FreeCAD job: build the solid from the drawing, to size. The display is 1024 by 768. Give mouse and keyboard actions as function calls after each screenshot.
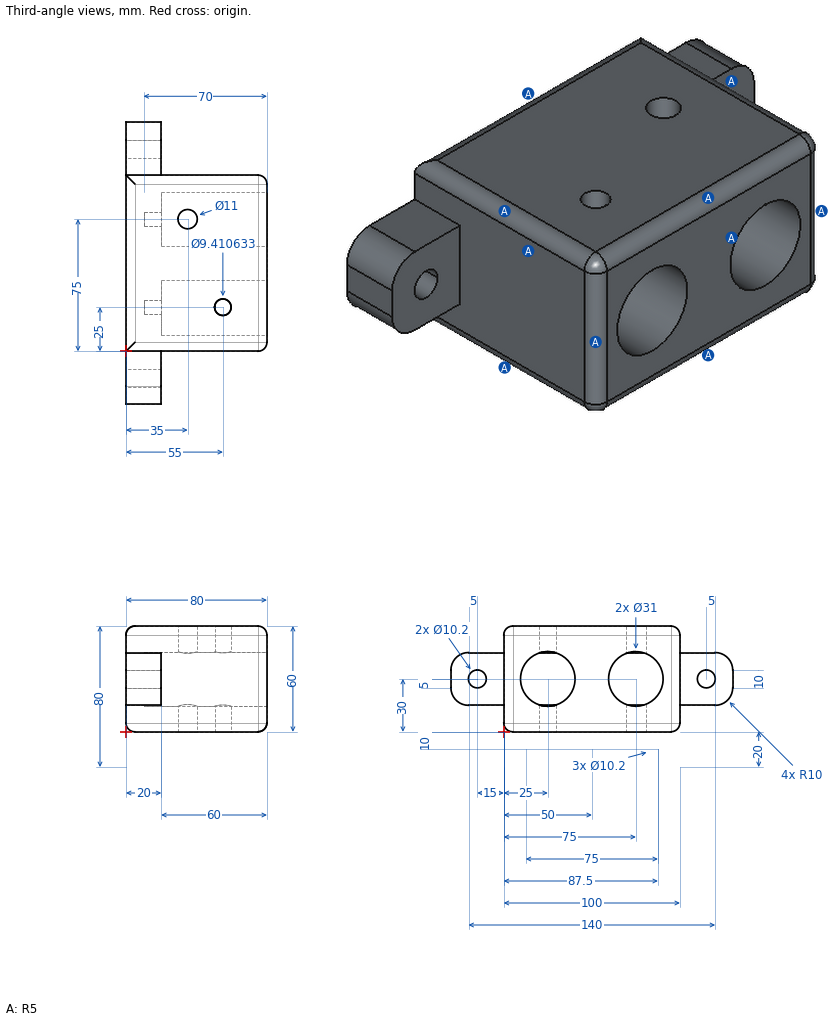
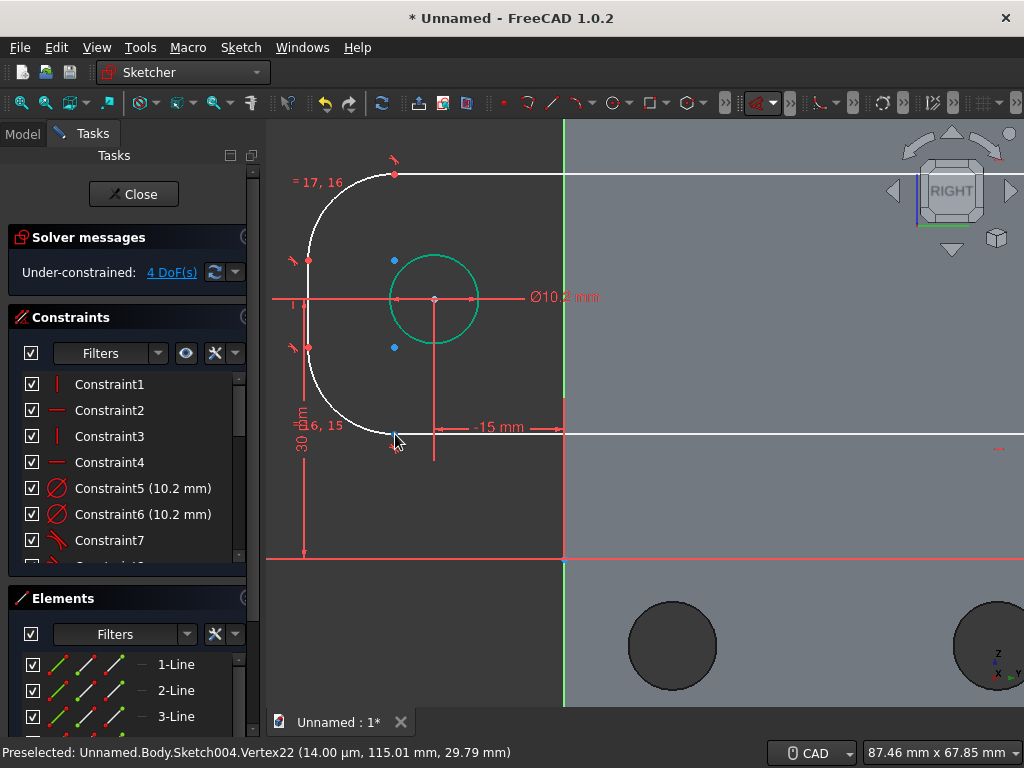
click(395, 434)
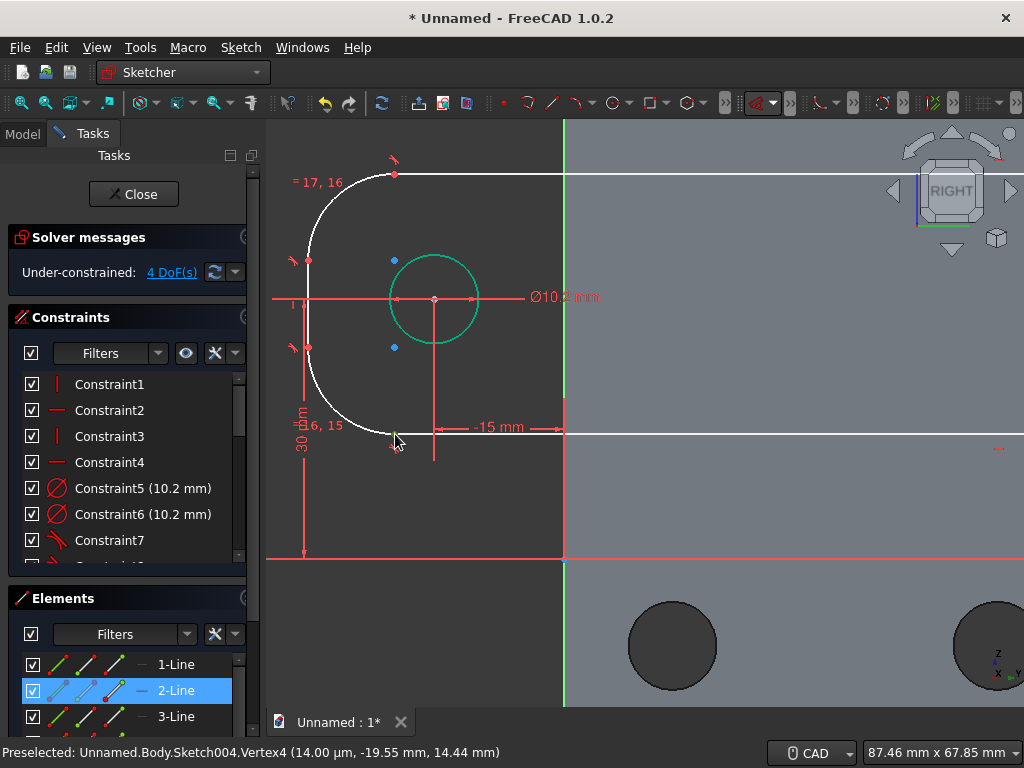
click(434, 299)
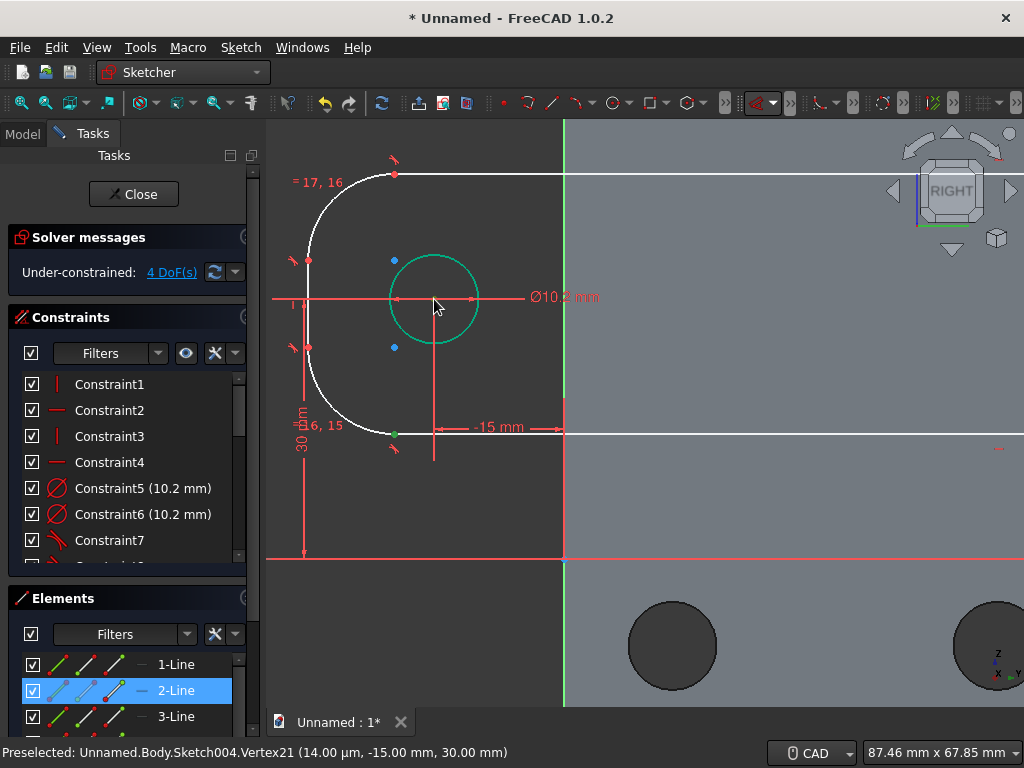
key(l)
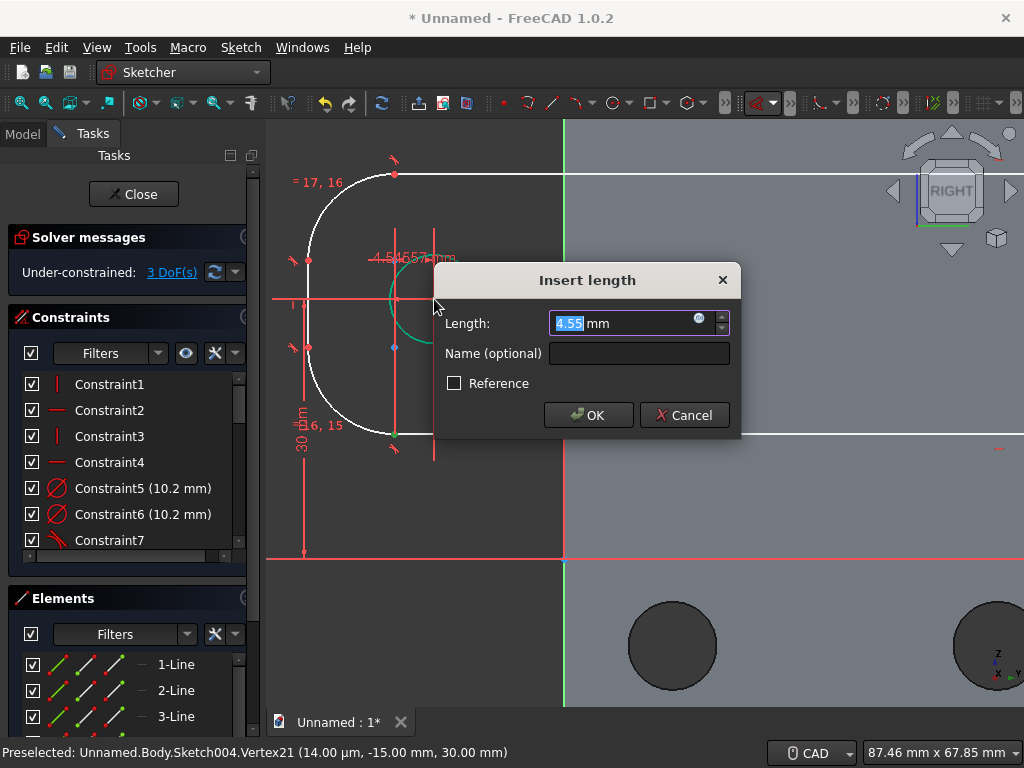
text(5)
key(Return)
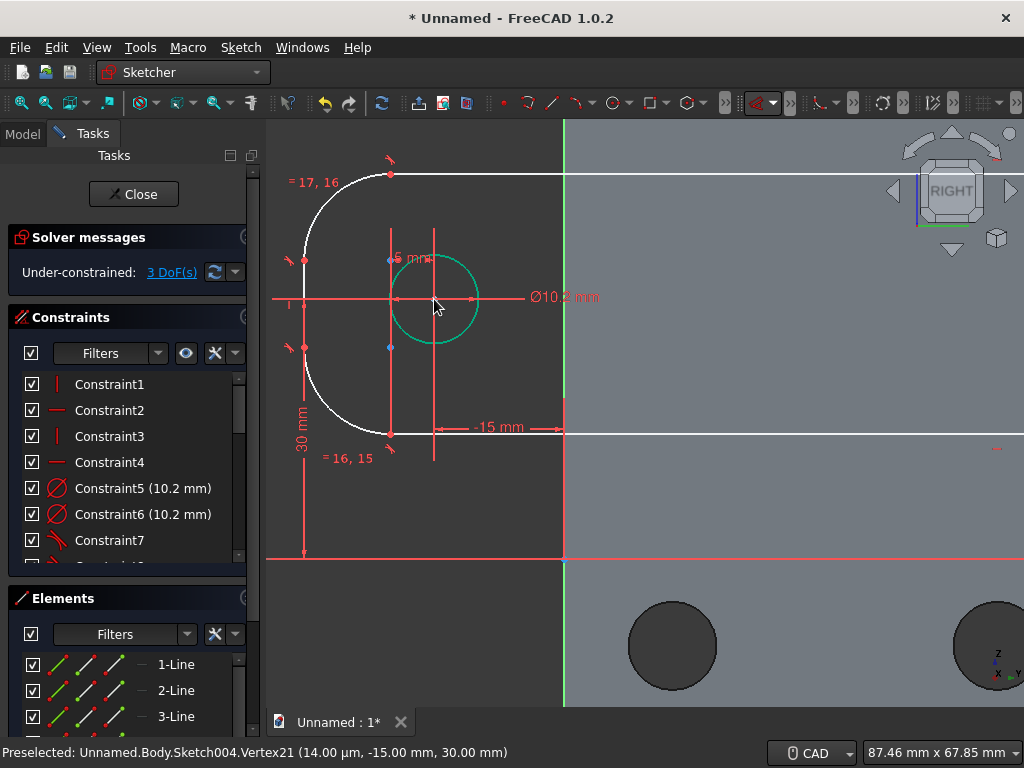
click(304, 347)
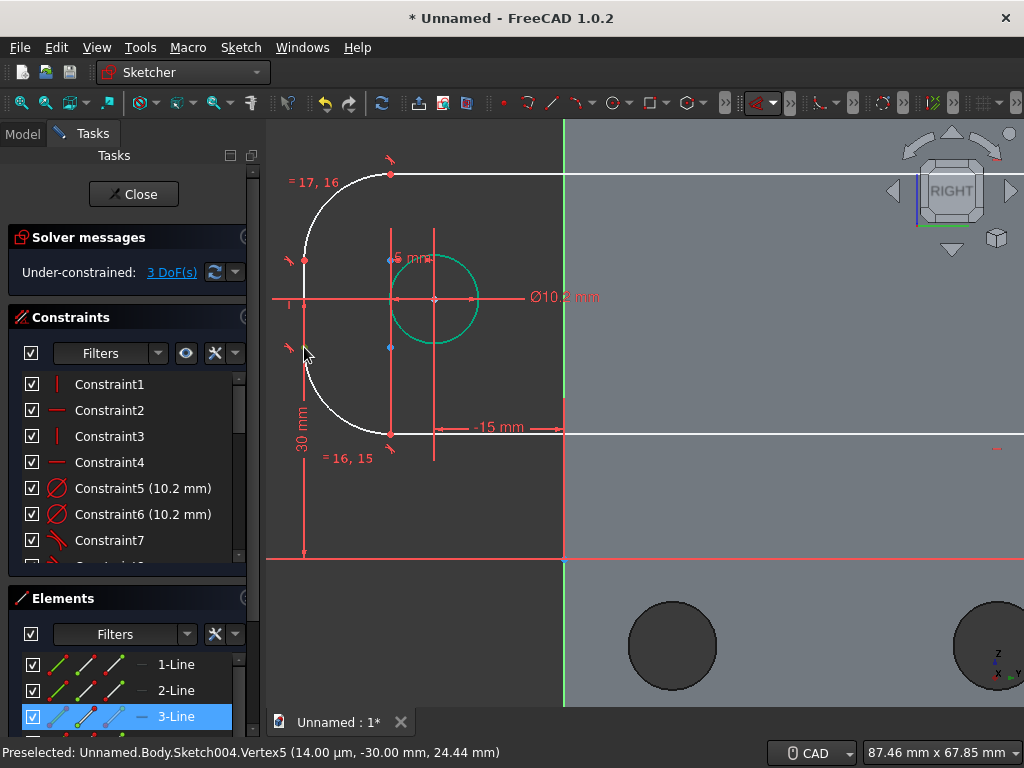
click(434, 299)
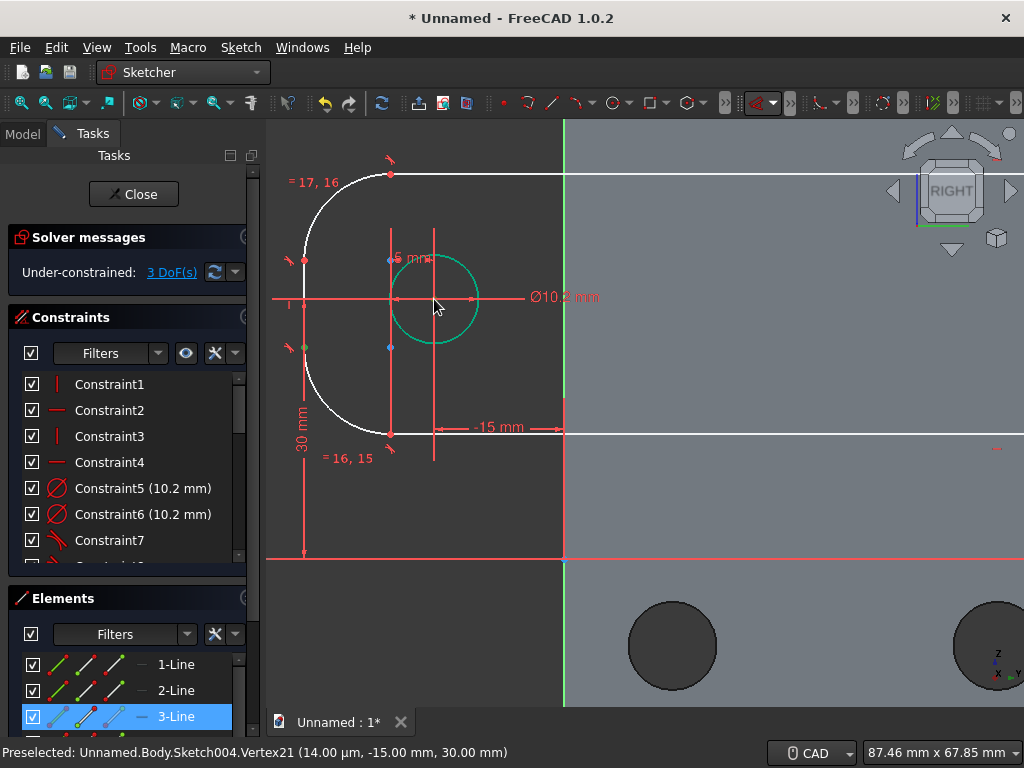
key(i)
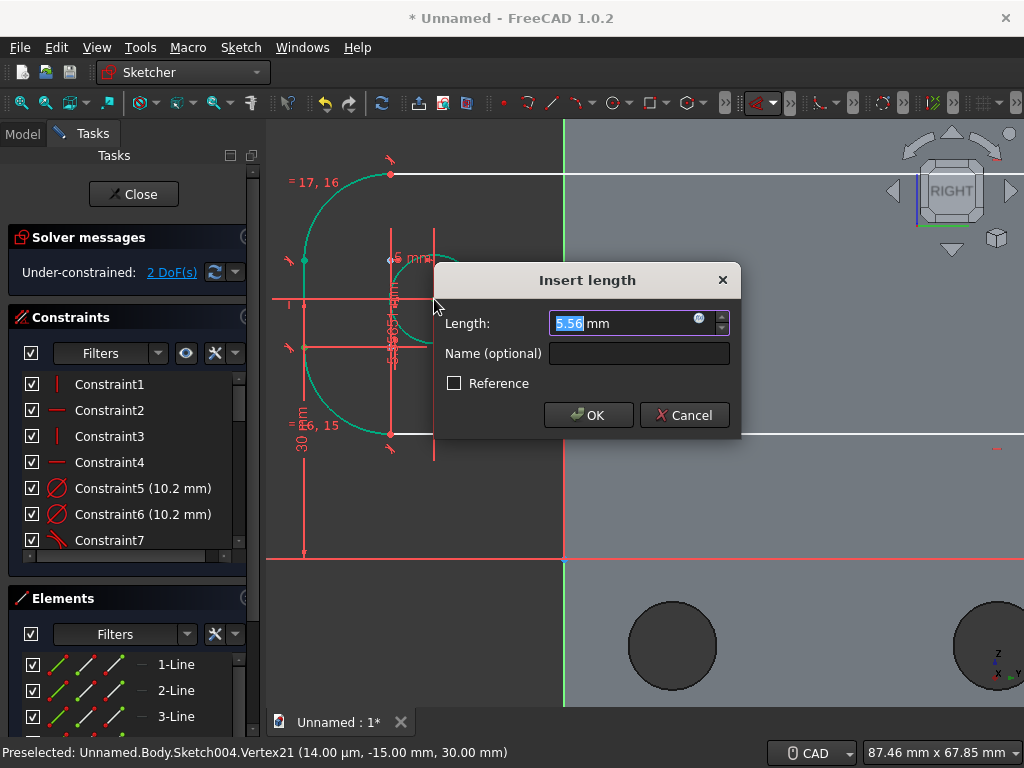
text(5)
key(Return)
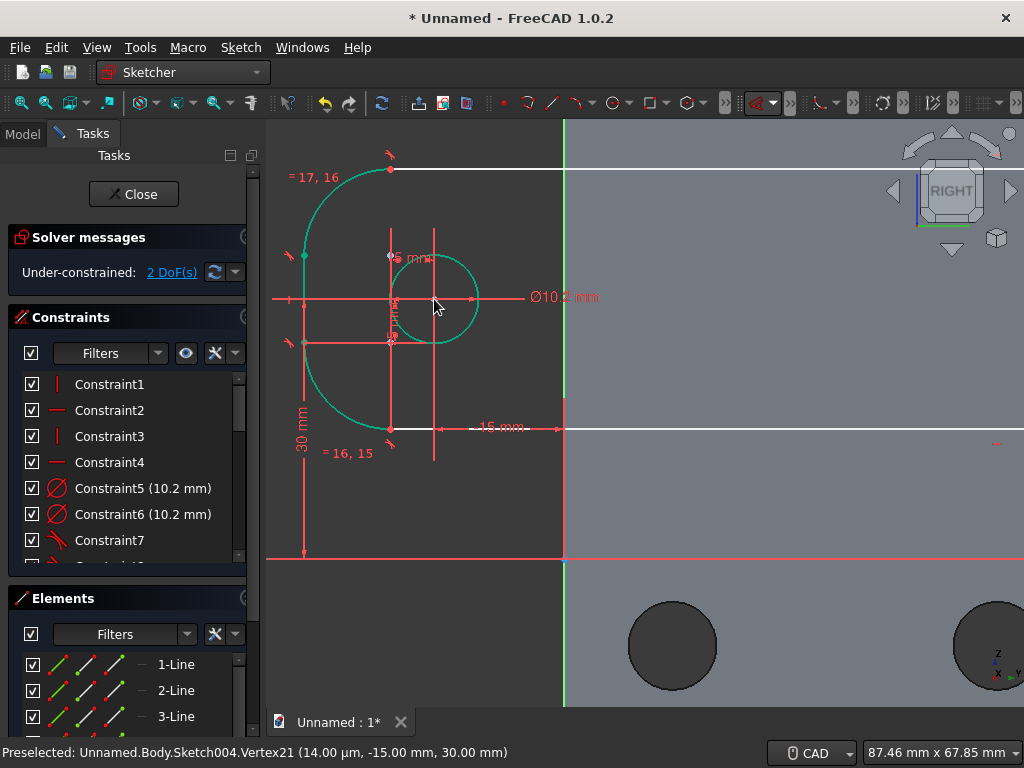
scroll(395, 434, down, 6)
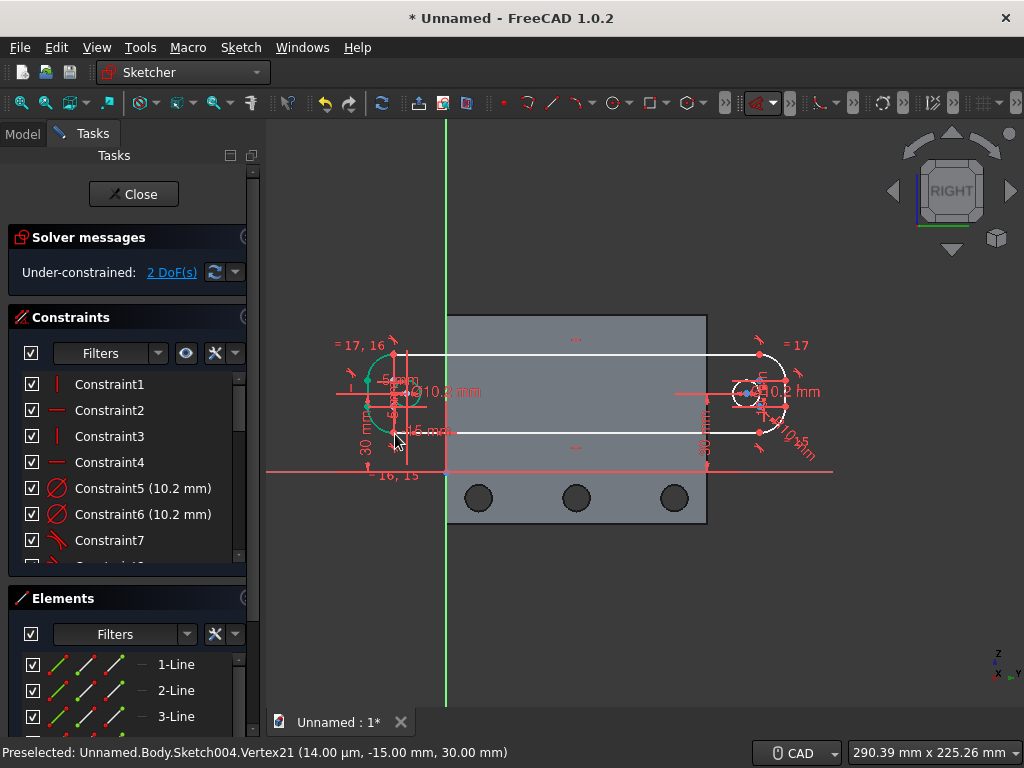
scroll(759, 433, up, 6)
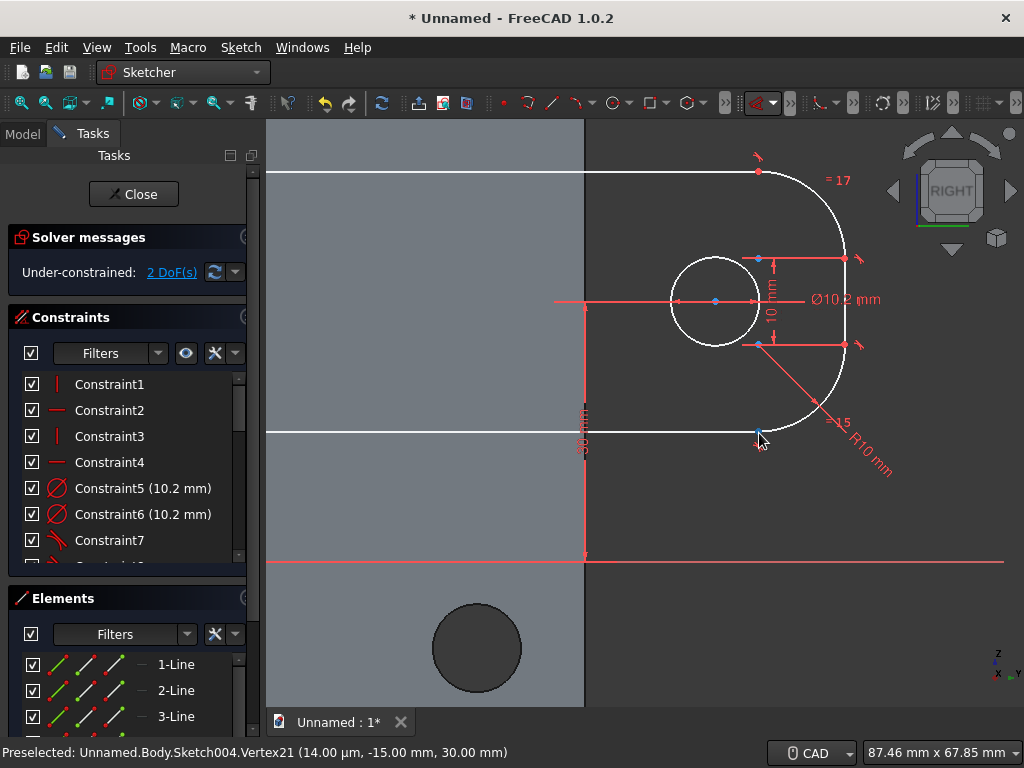
click(758, 432)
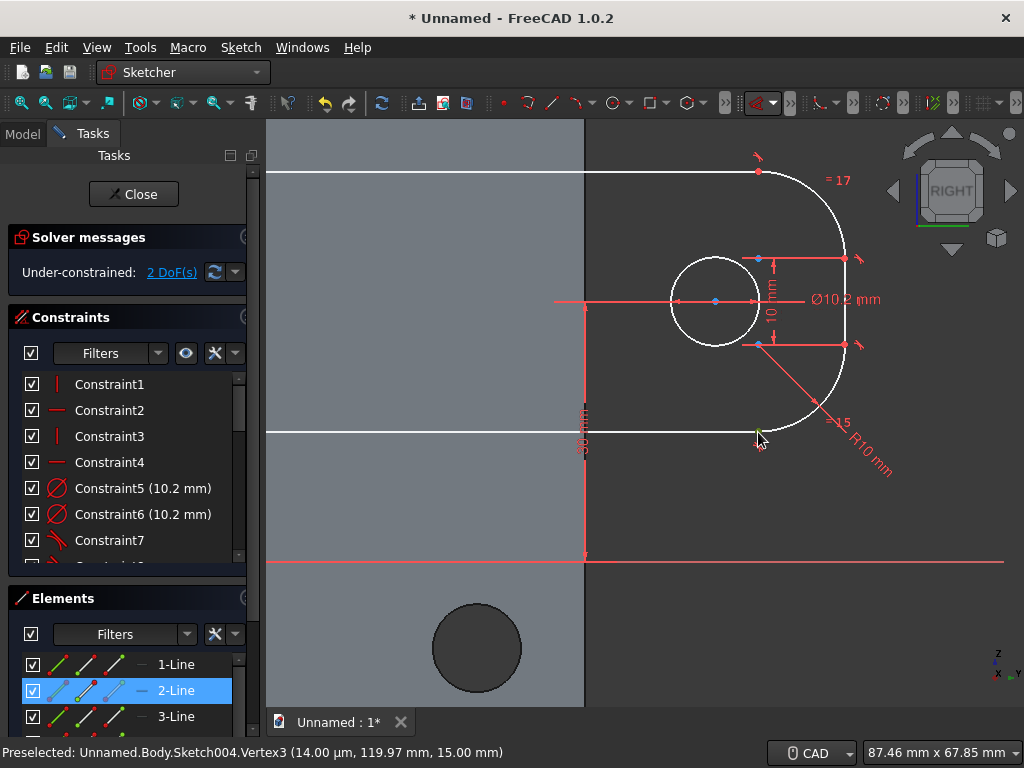
click(715, 302)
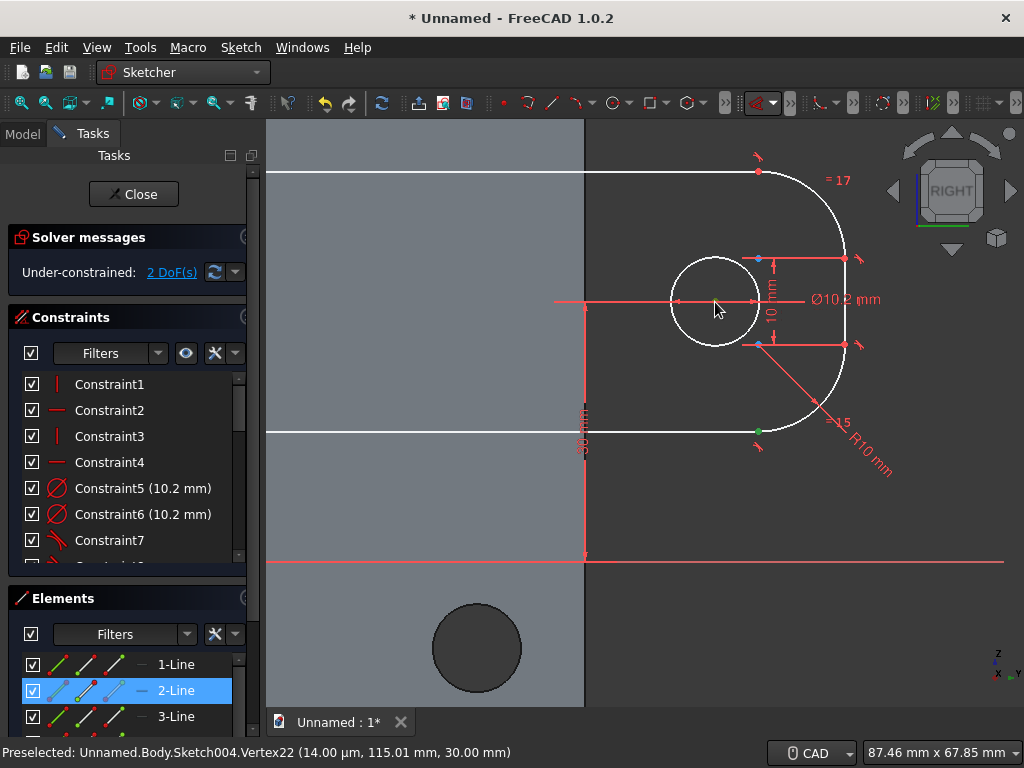
key(l)